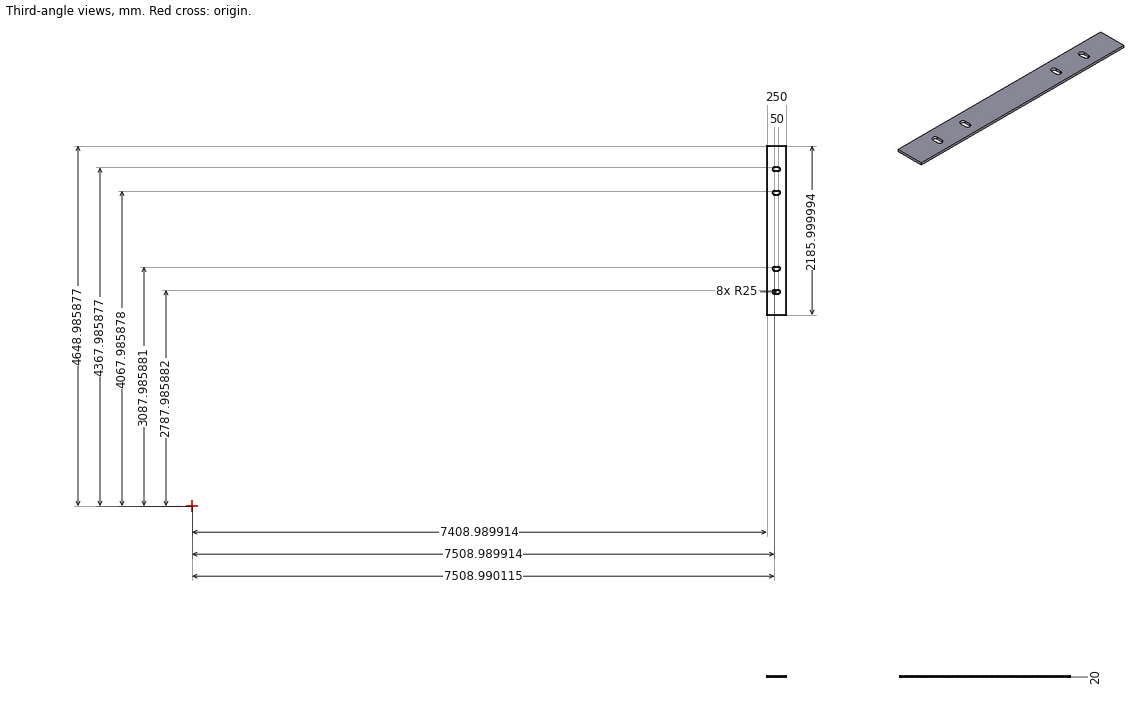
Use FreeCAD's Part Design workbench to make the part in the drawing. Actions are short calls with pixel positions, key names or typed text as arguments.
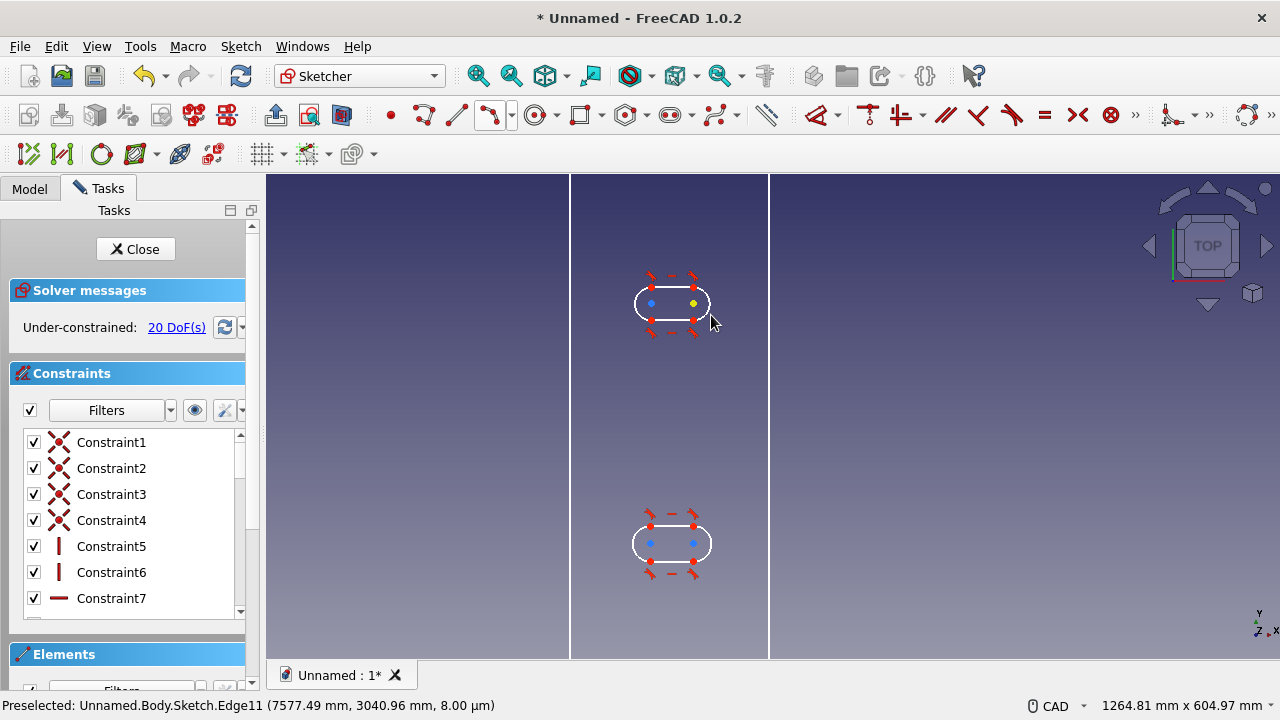
click(706, 314)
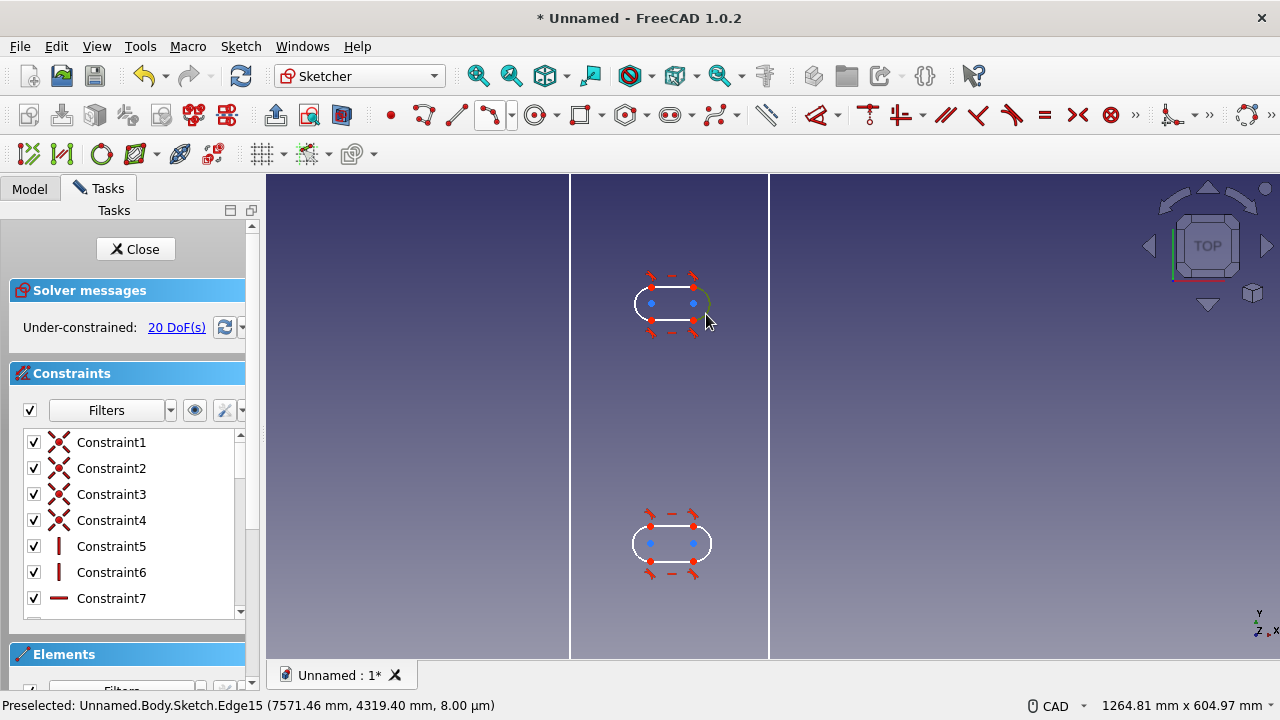
click(708, 554)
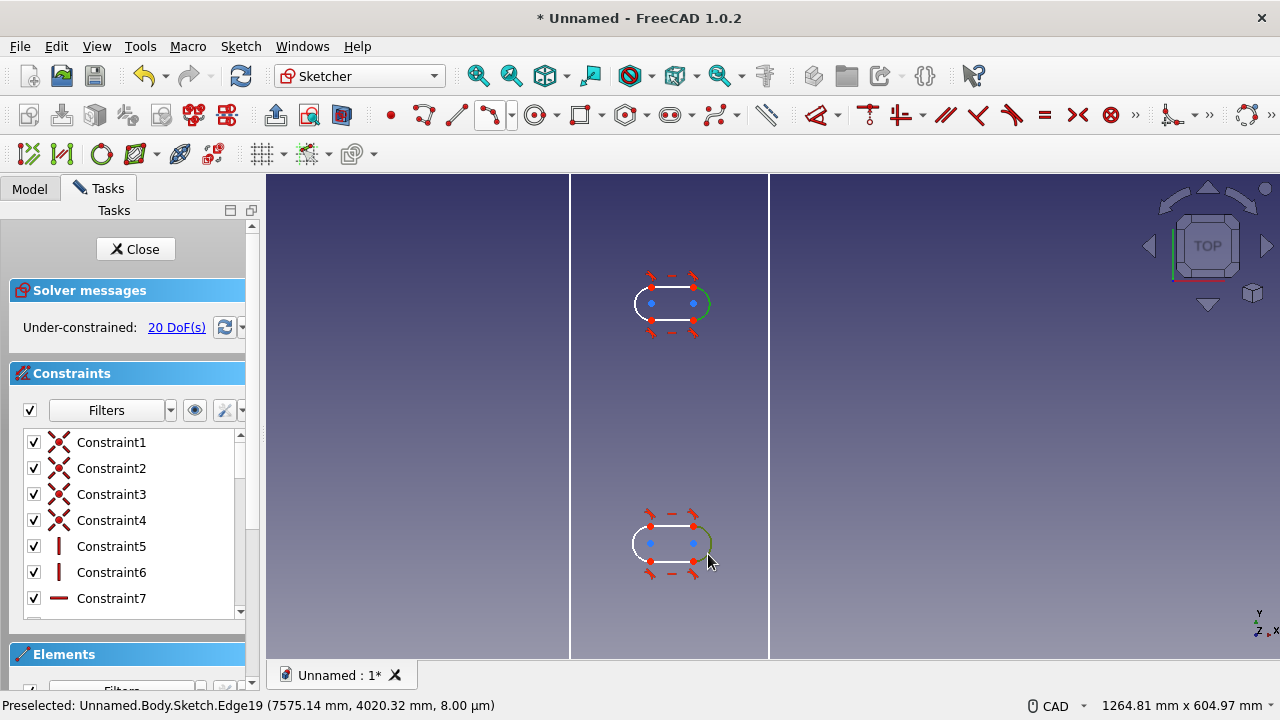
key(e)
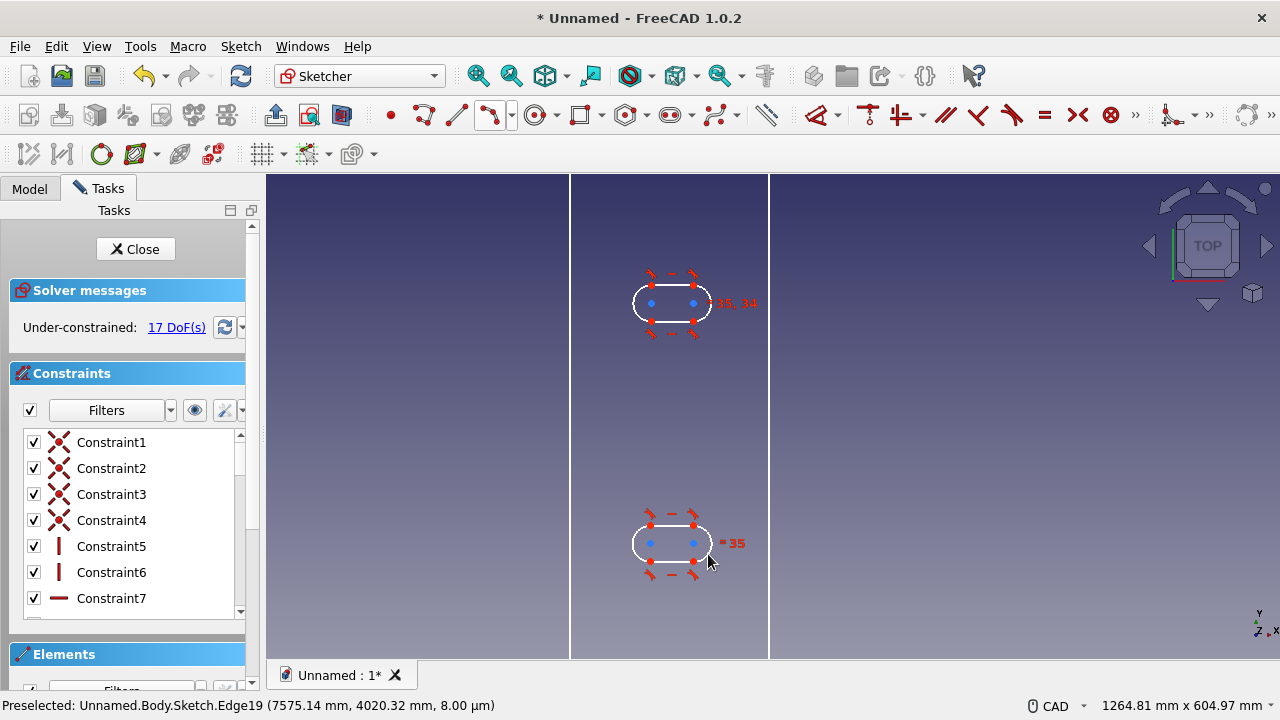
key(d)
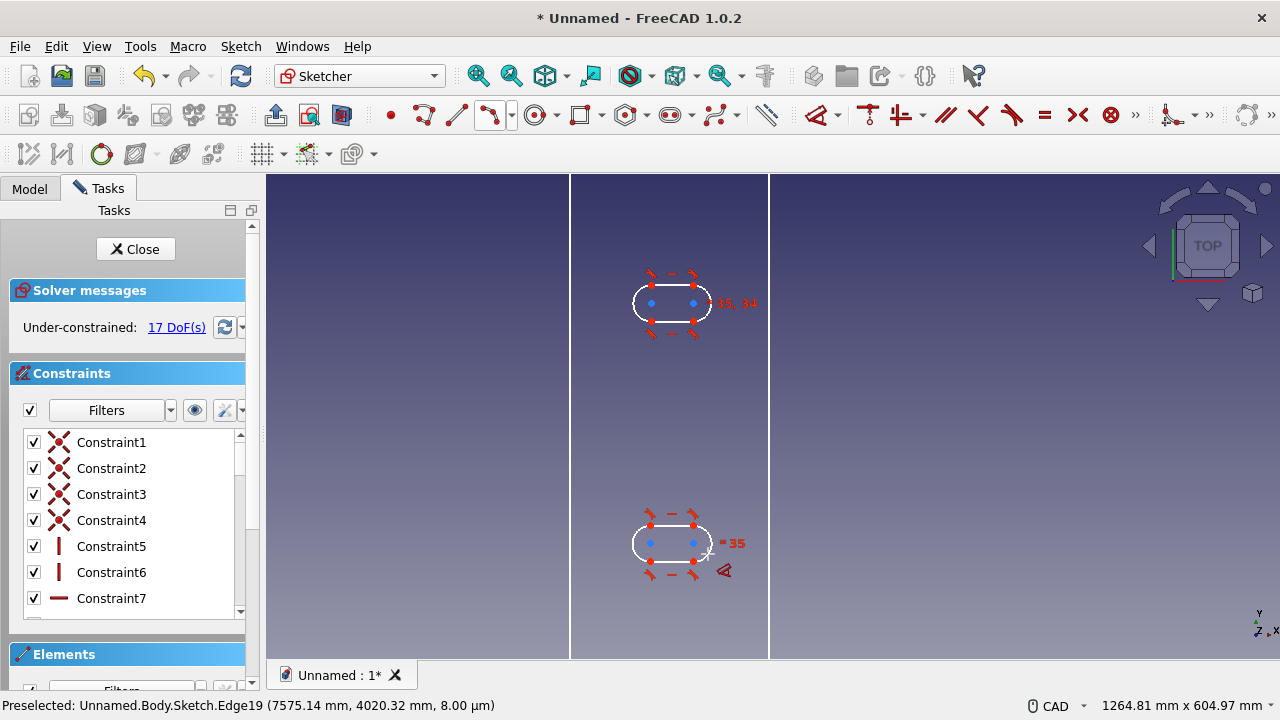
scroll(711, 315, down, 9)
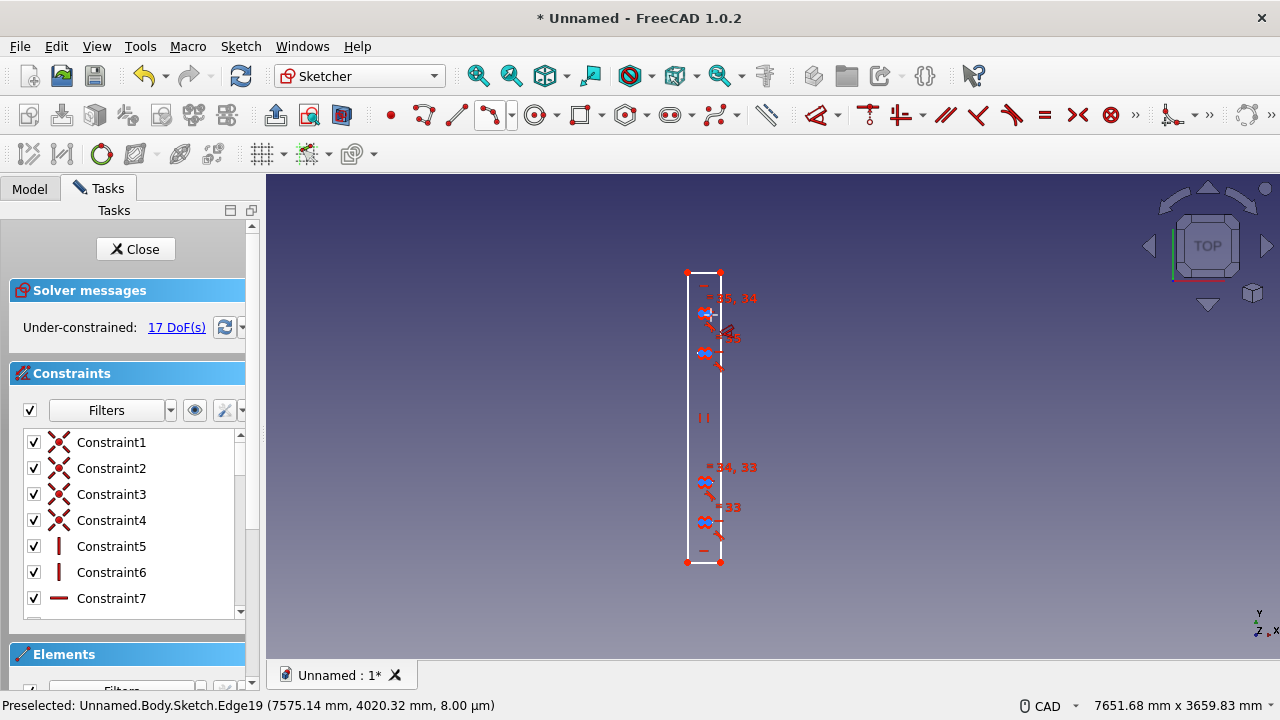
scroll(711, 524, up, 13)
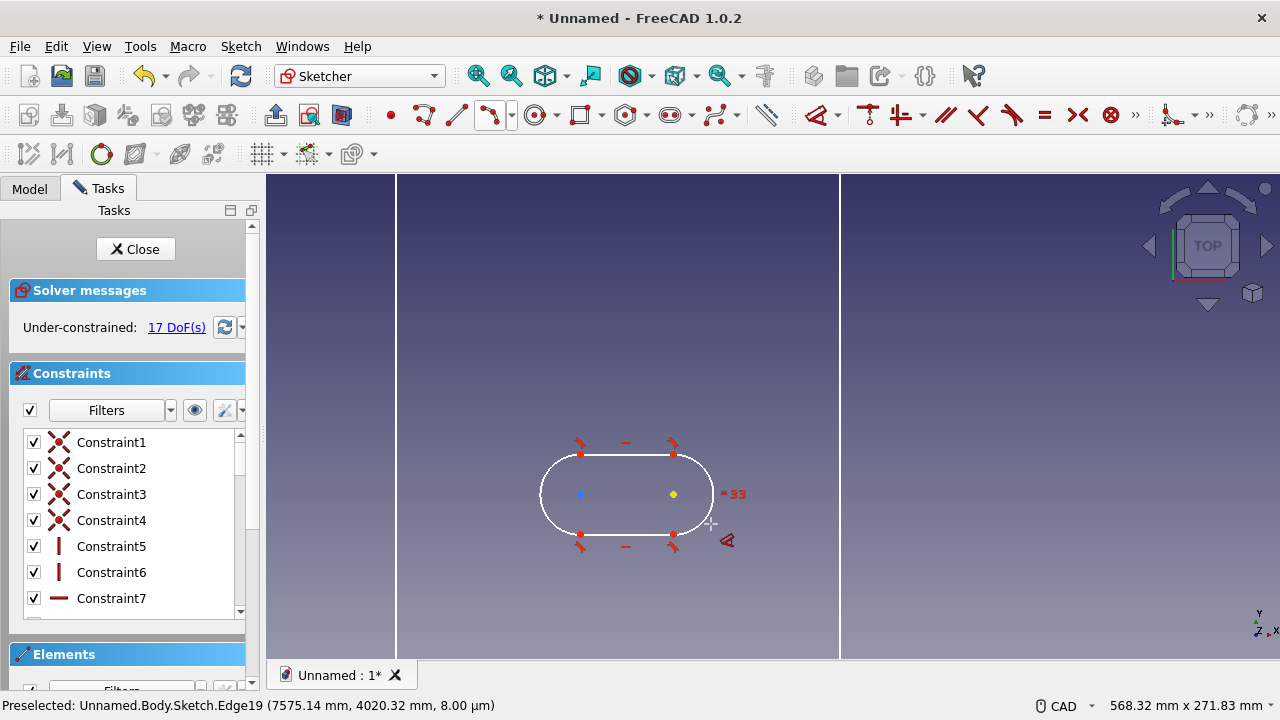
click(706, 518)
click(732, 537)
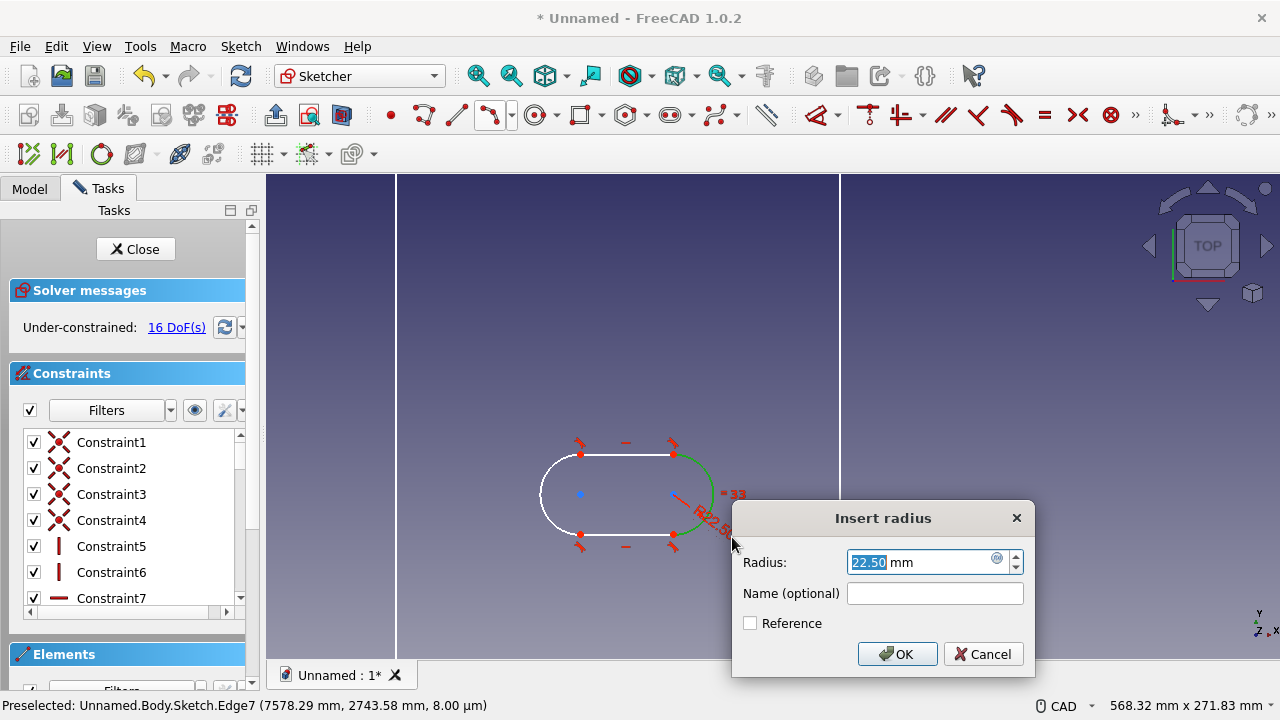
text(25)
key(Return)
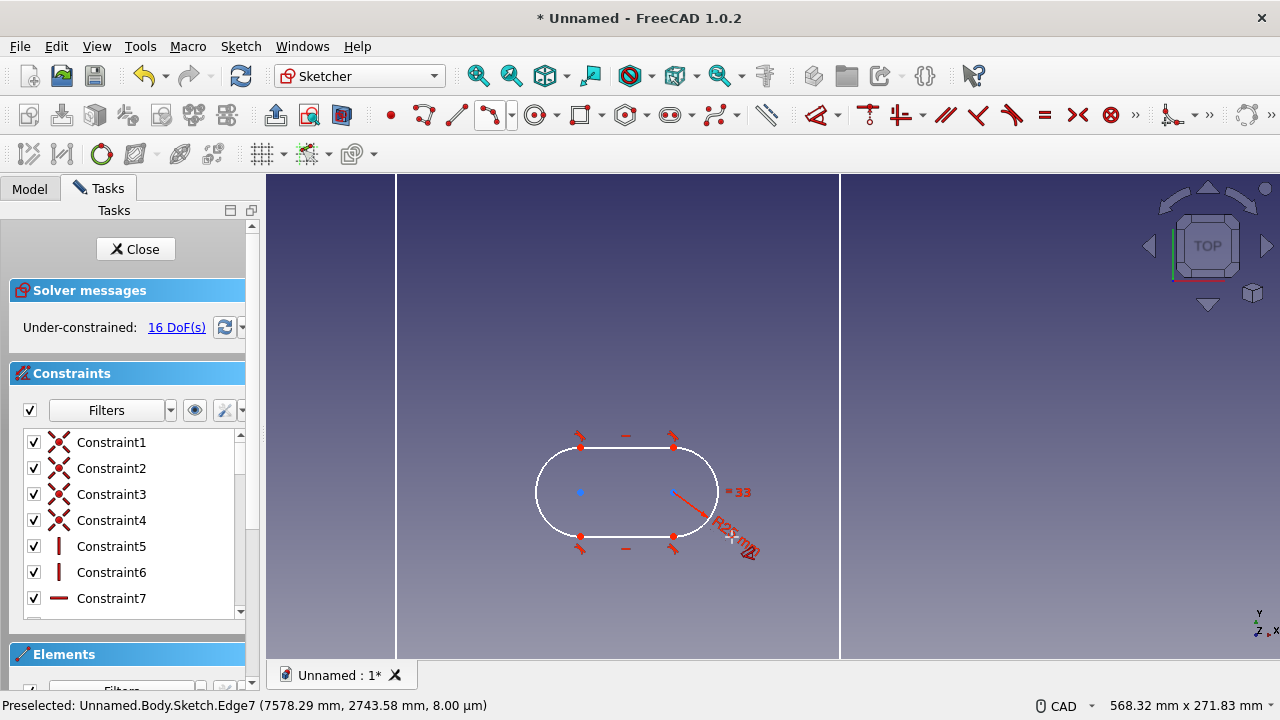
click(645, 537)
click(627, 571)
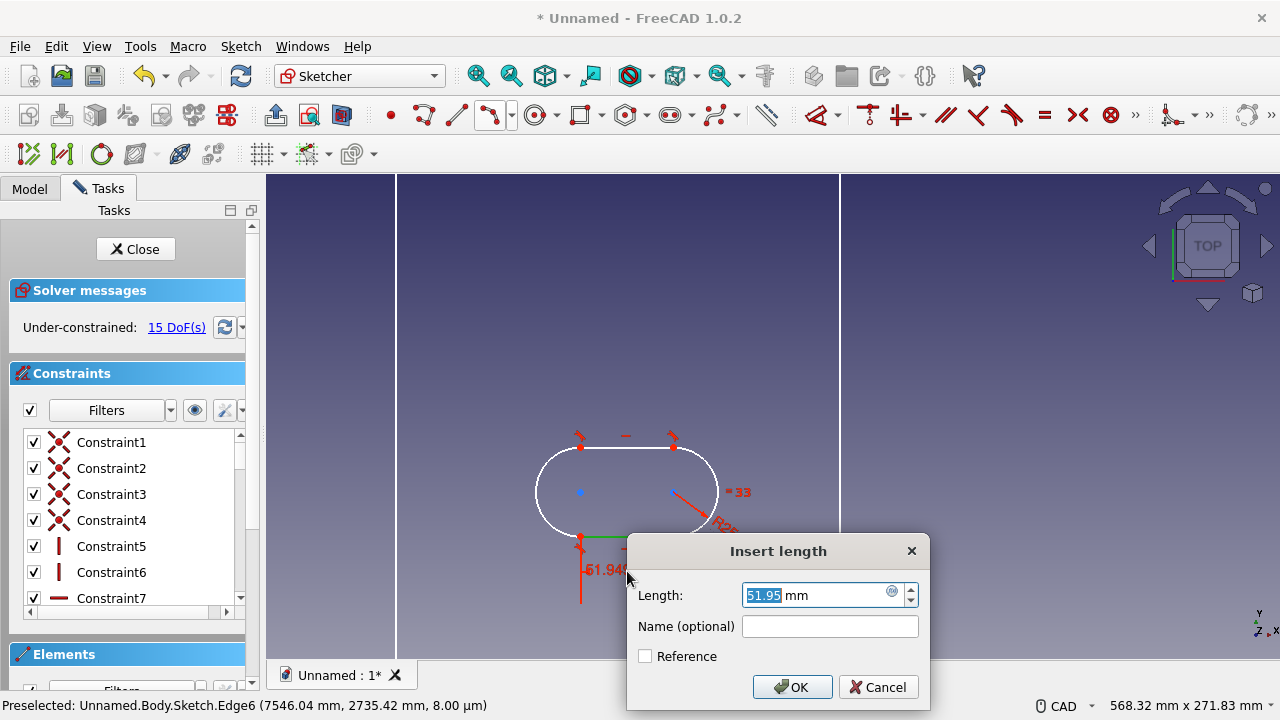
text(50)
key(Return)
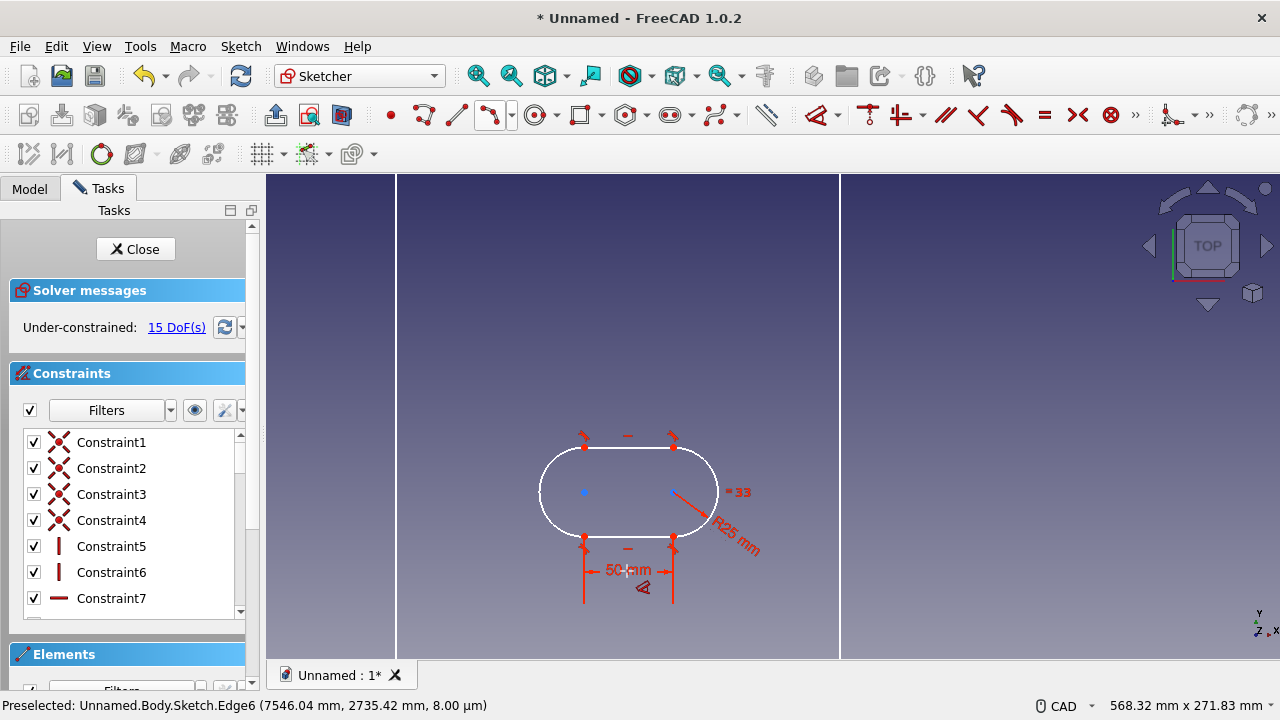
scroll(711, 524, down, 13)